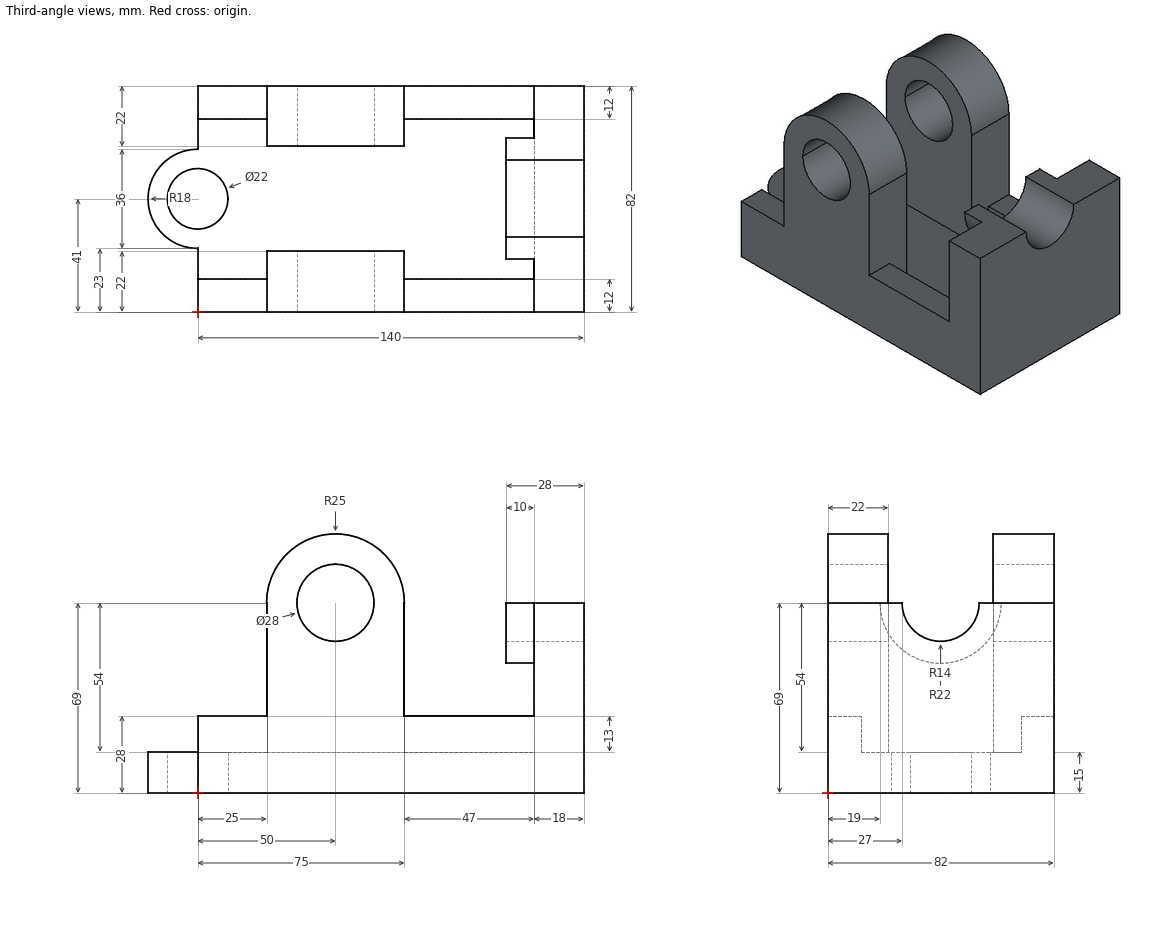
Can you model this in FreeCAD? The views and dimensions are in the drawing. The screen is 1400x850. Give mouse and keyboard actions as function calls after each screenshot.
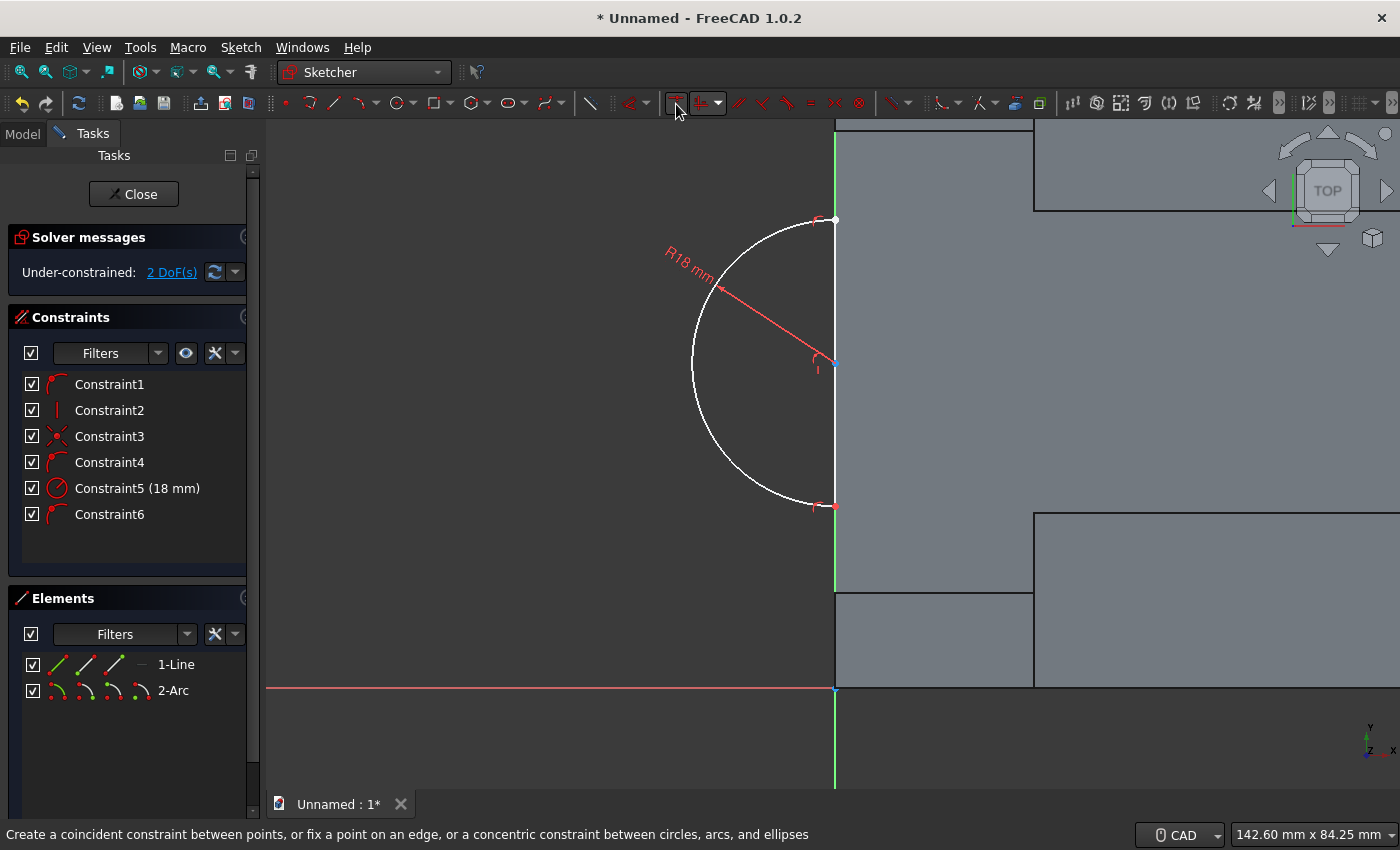
click(630, 104)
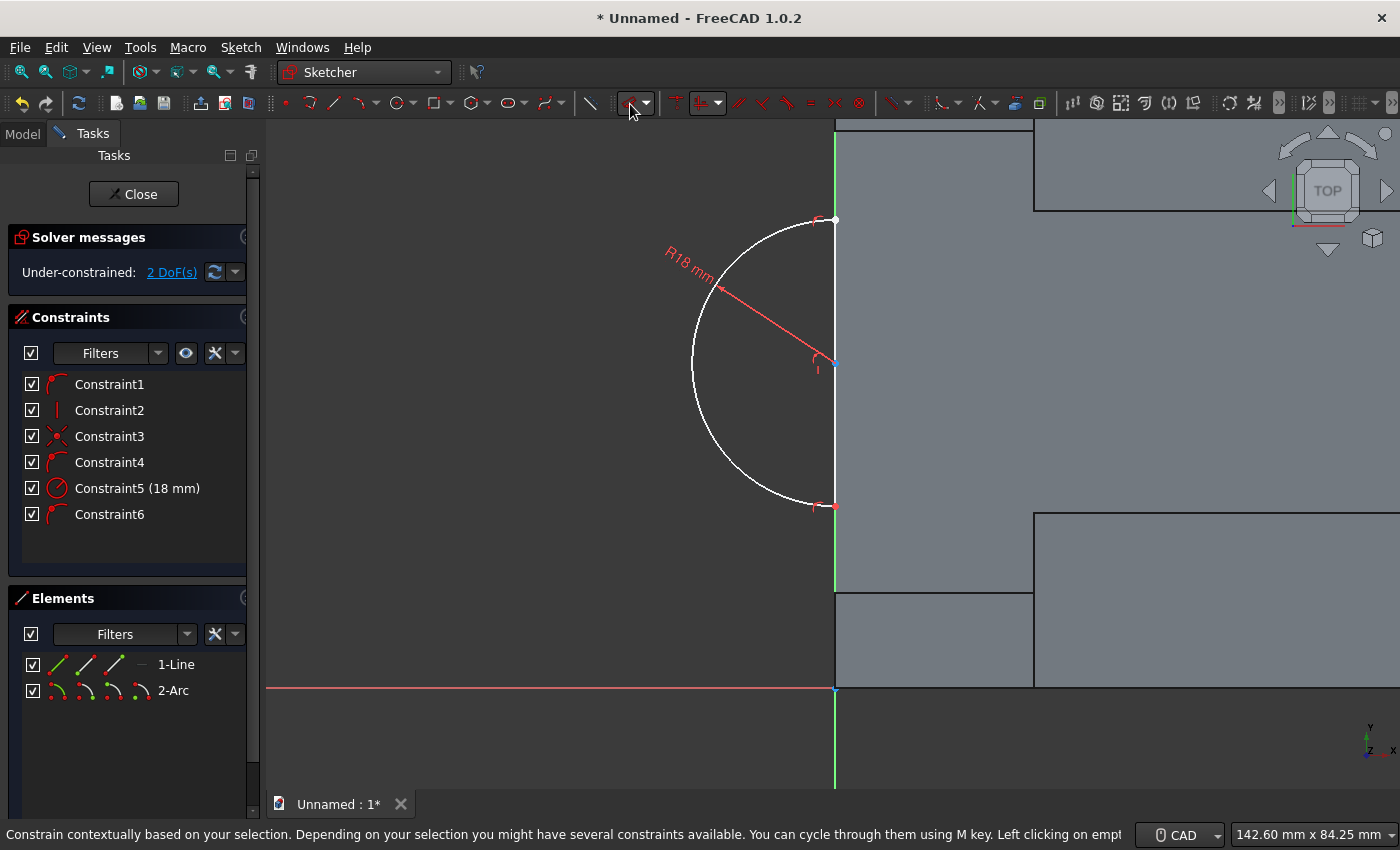
click(835, 420)
click(869, 363)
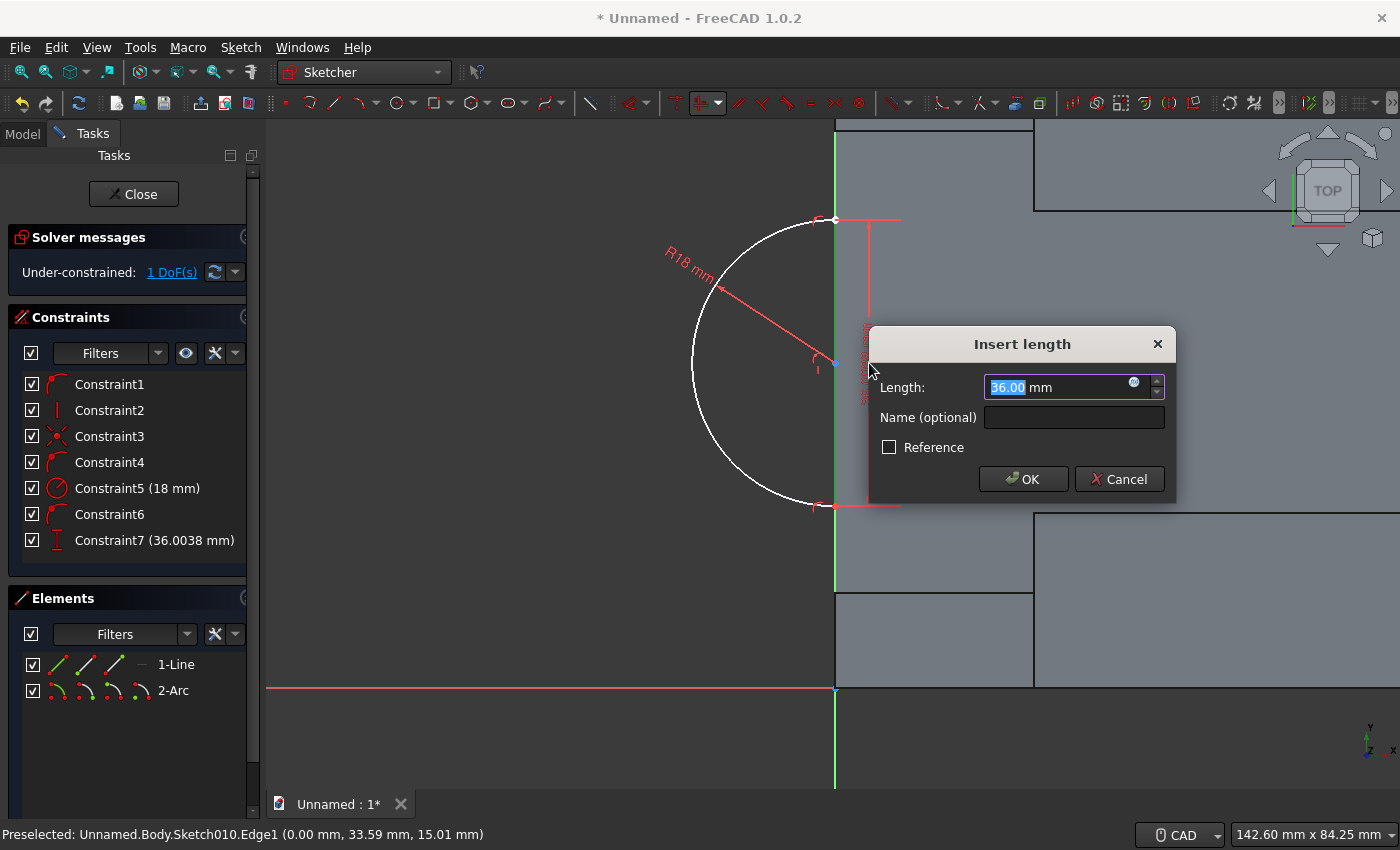
text(36)
key(Return)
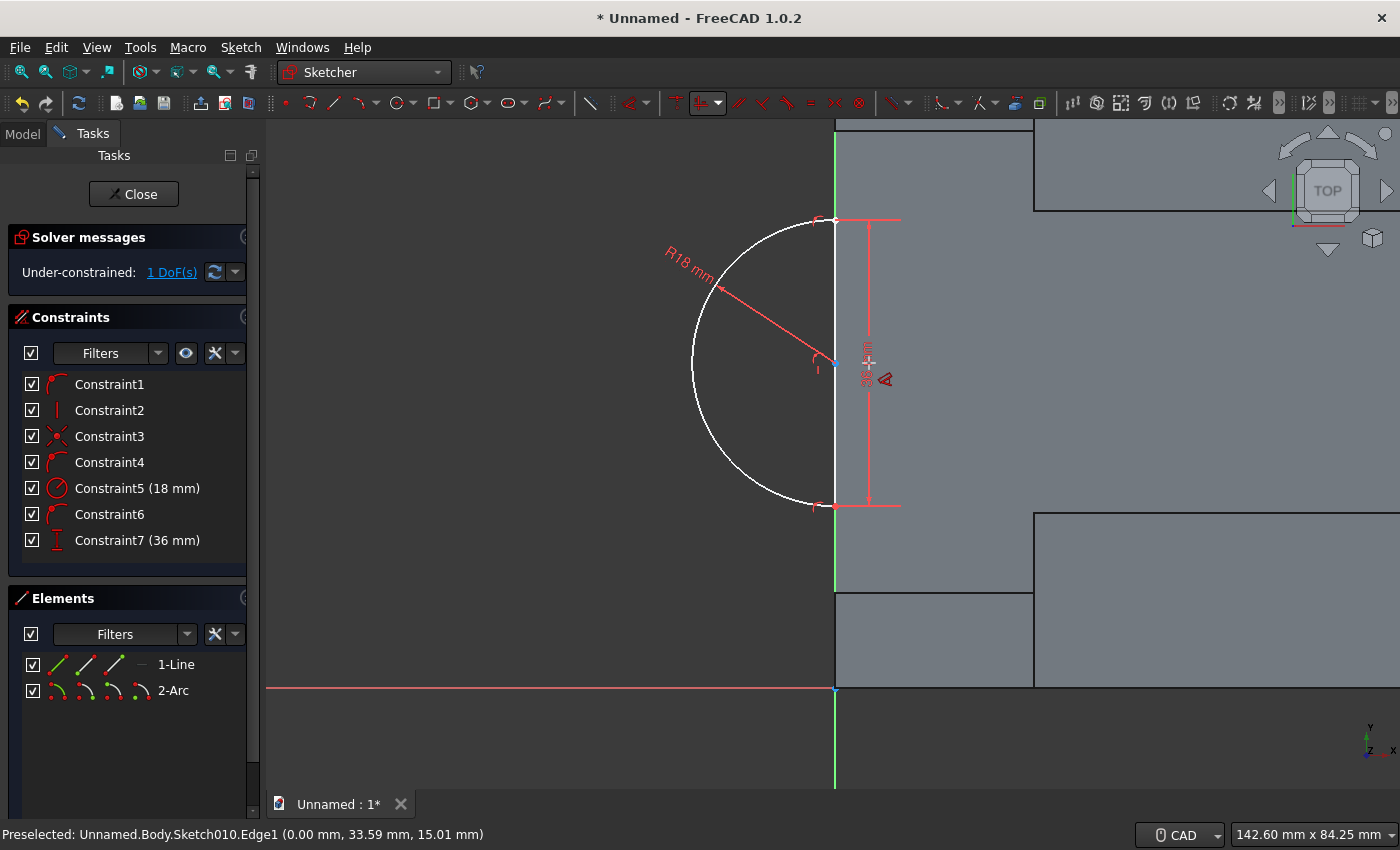
click(835, 506)
click(869, 597)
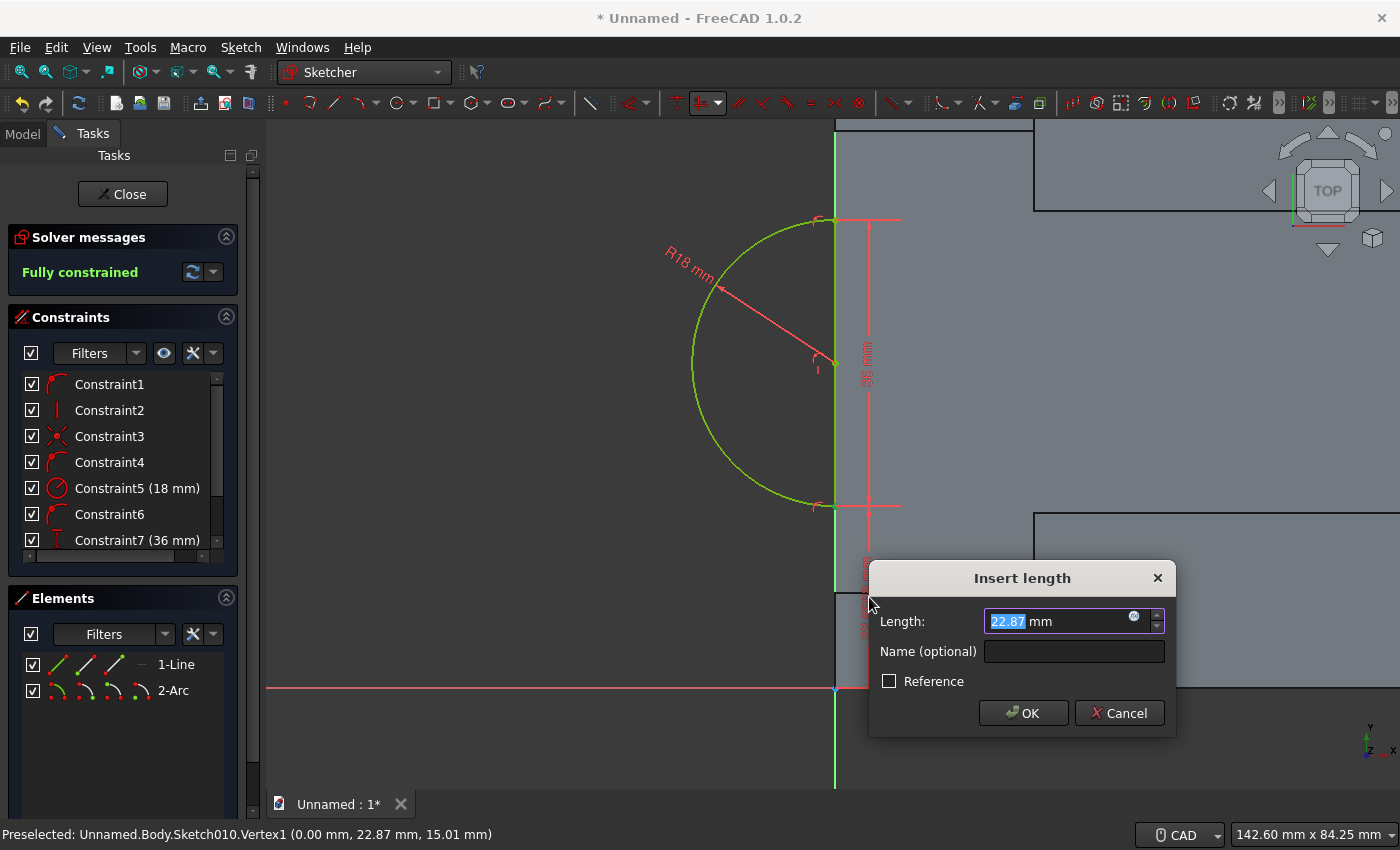
text(23)
key(Return)
key(Escape)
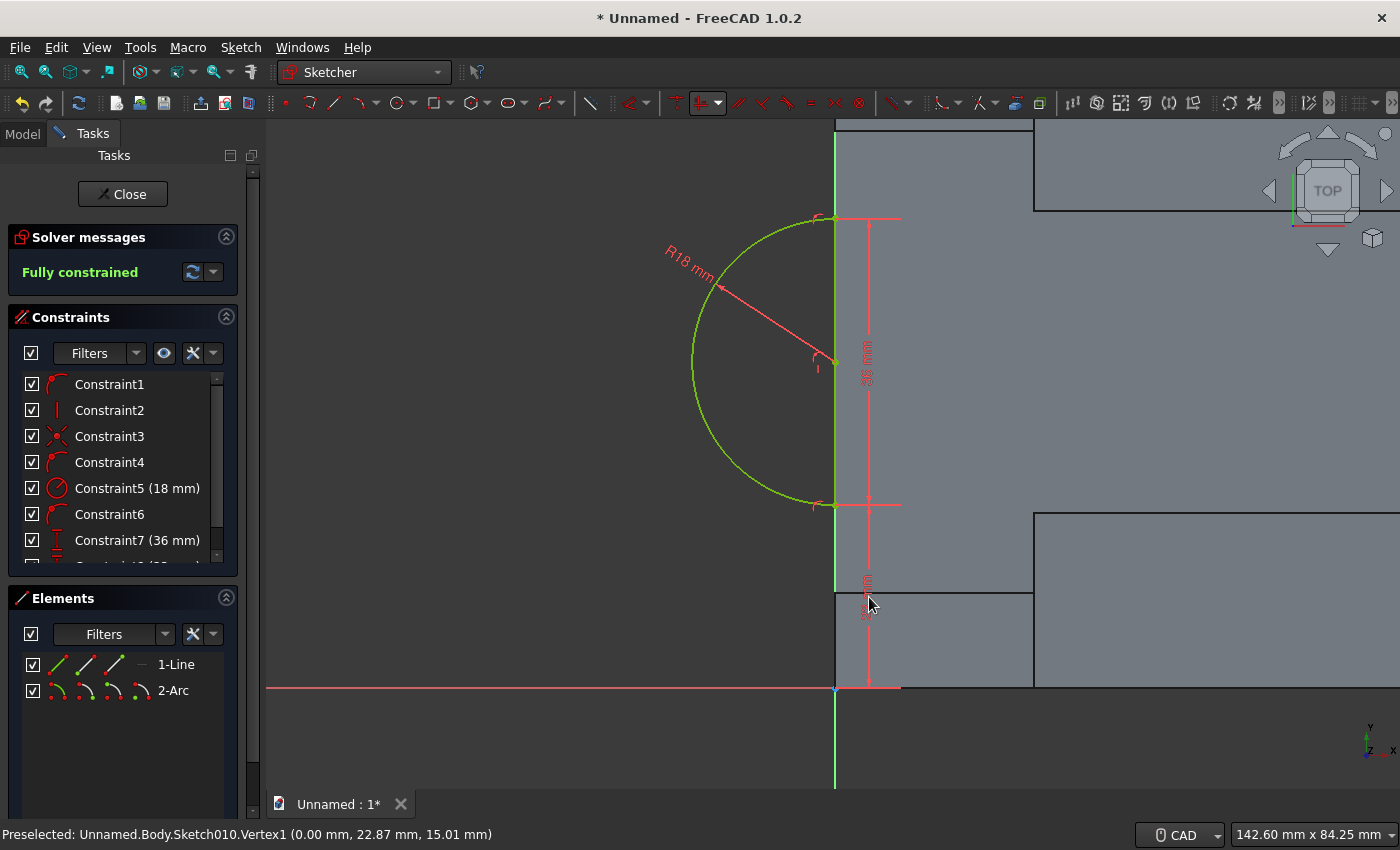
click(123, 194)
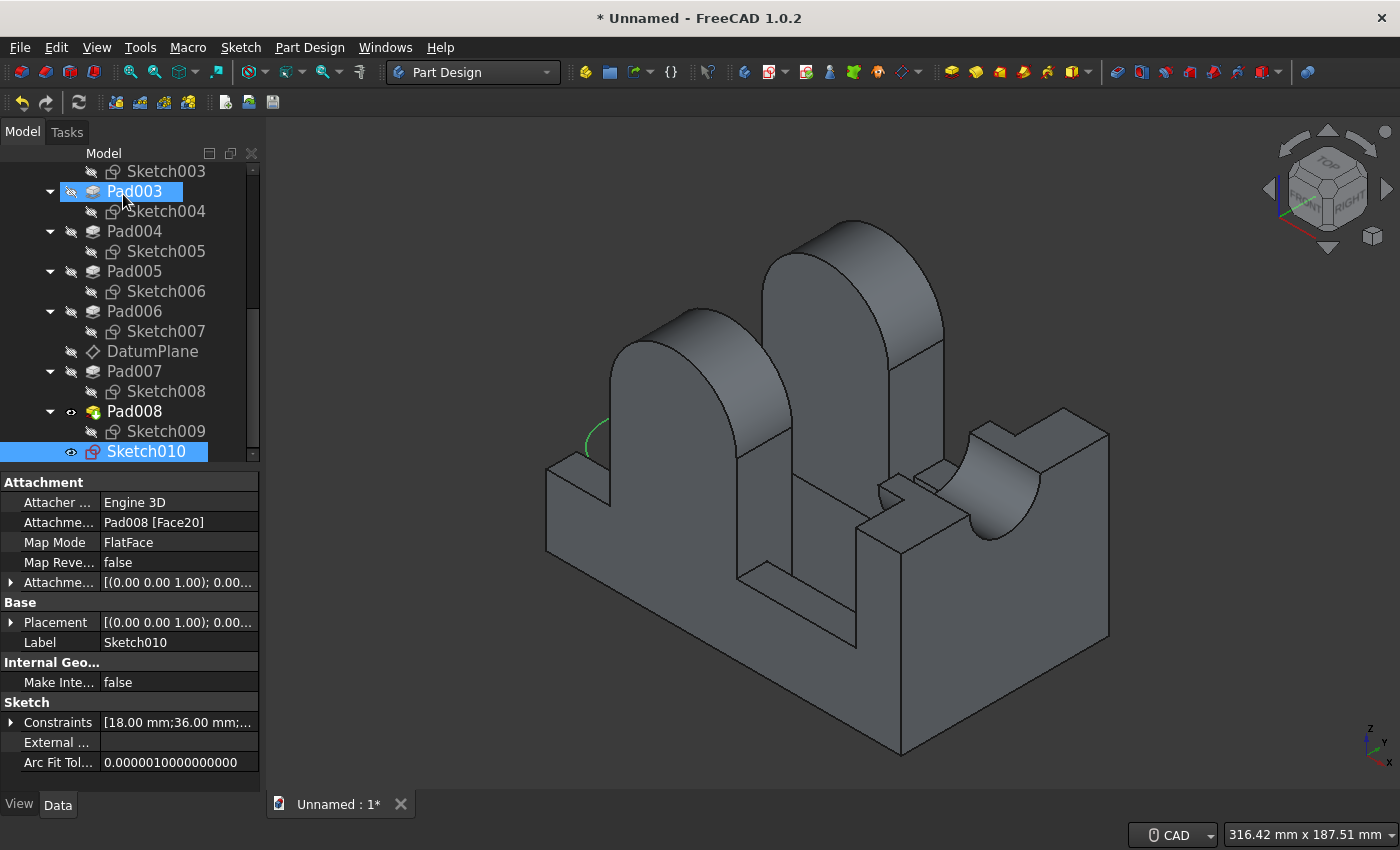
click(952, 72)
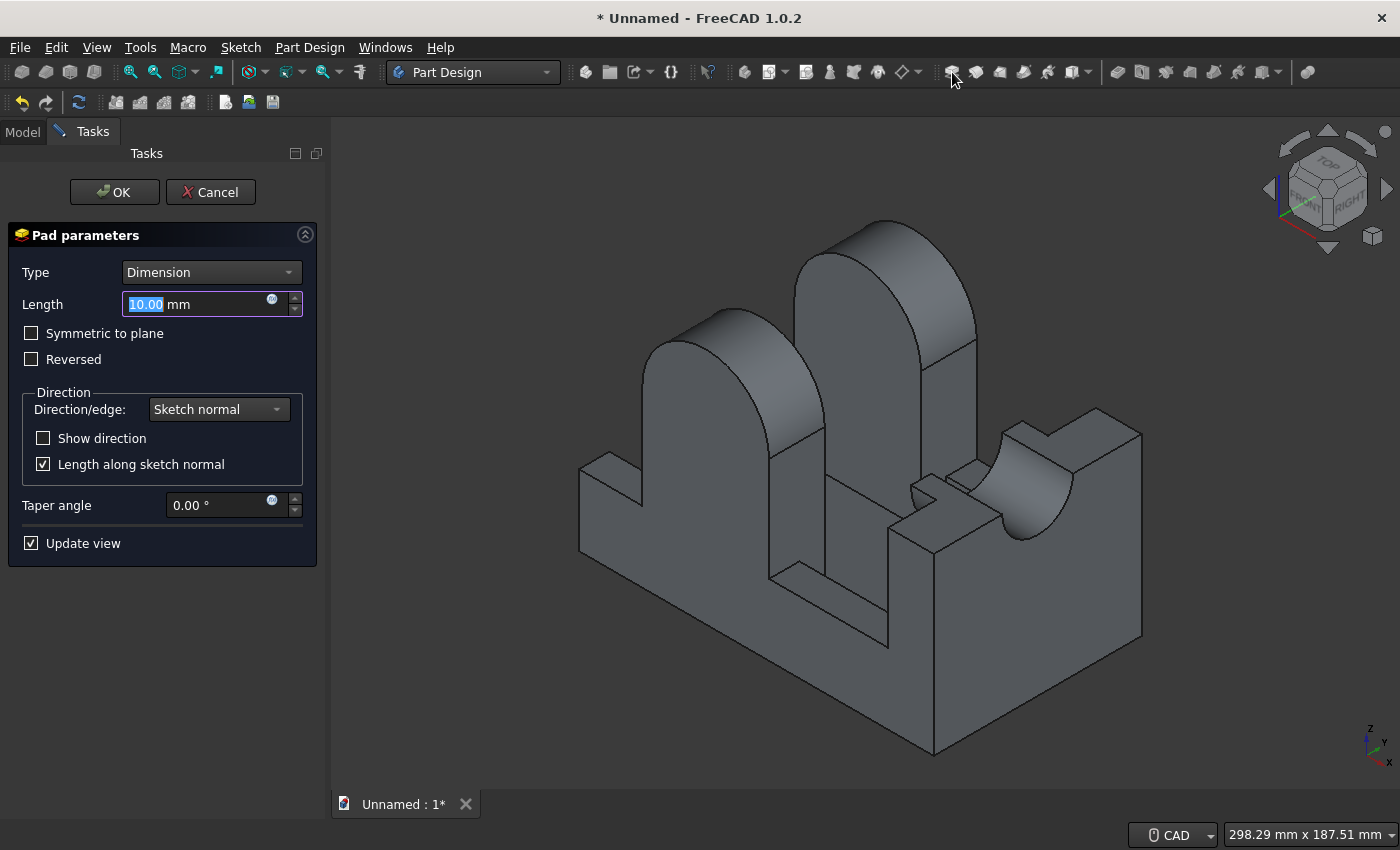
text(15)
key(Tab)